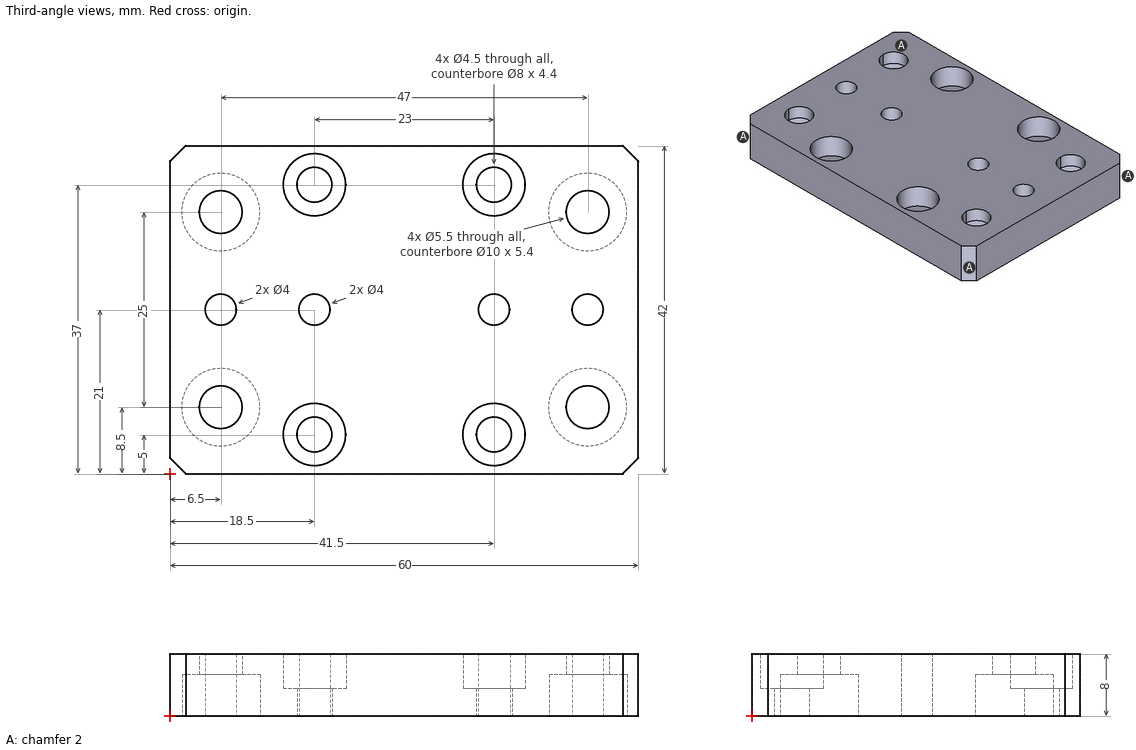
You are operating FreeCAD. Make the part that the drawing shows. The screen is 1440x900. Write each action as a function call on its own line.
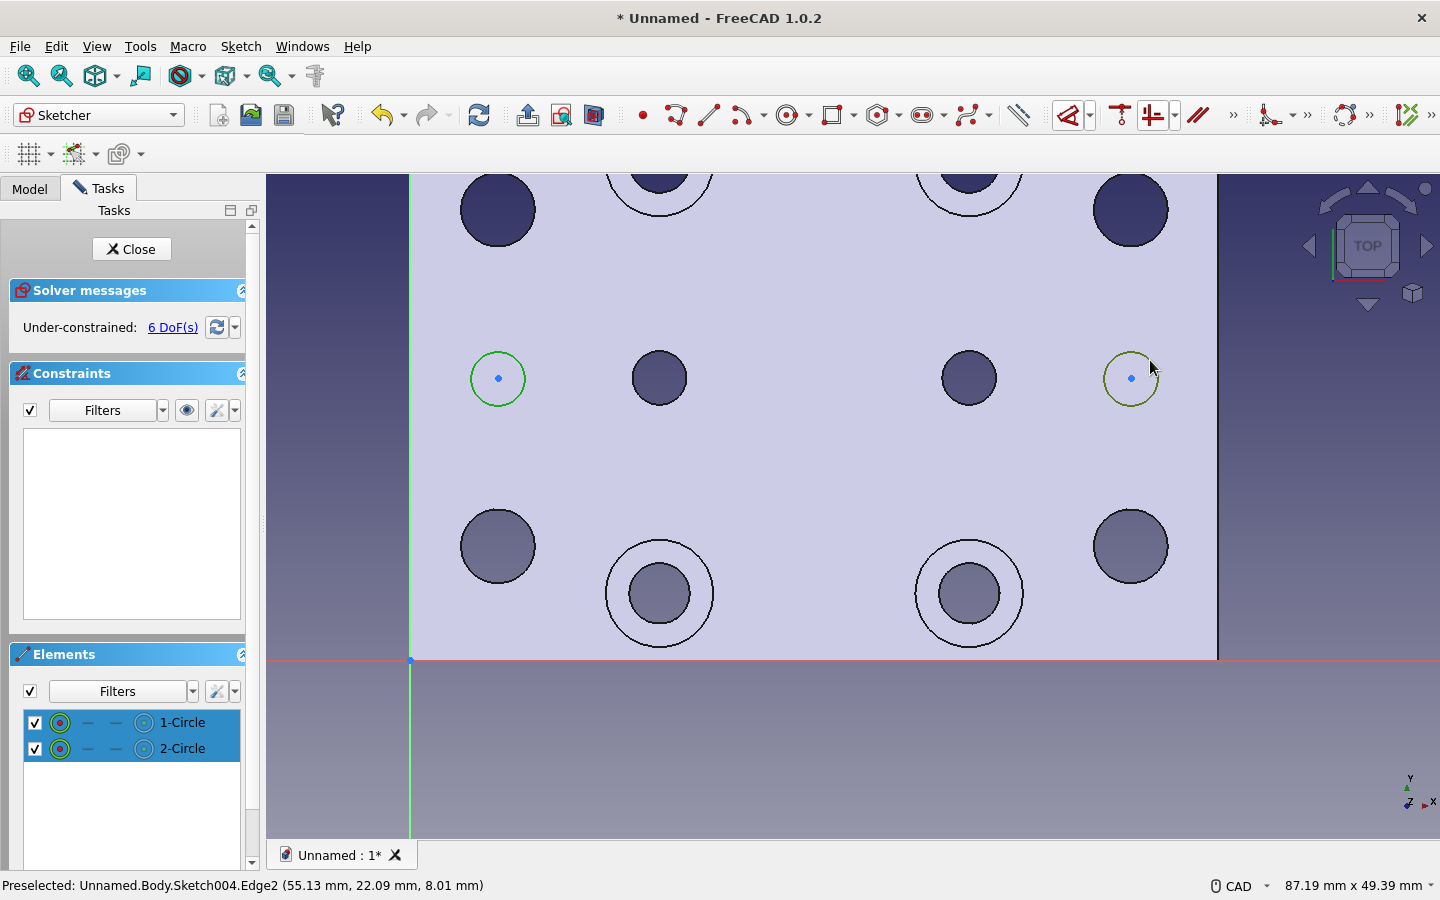
key(e)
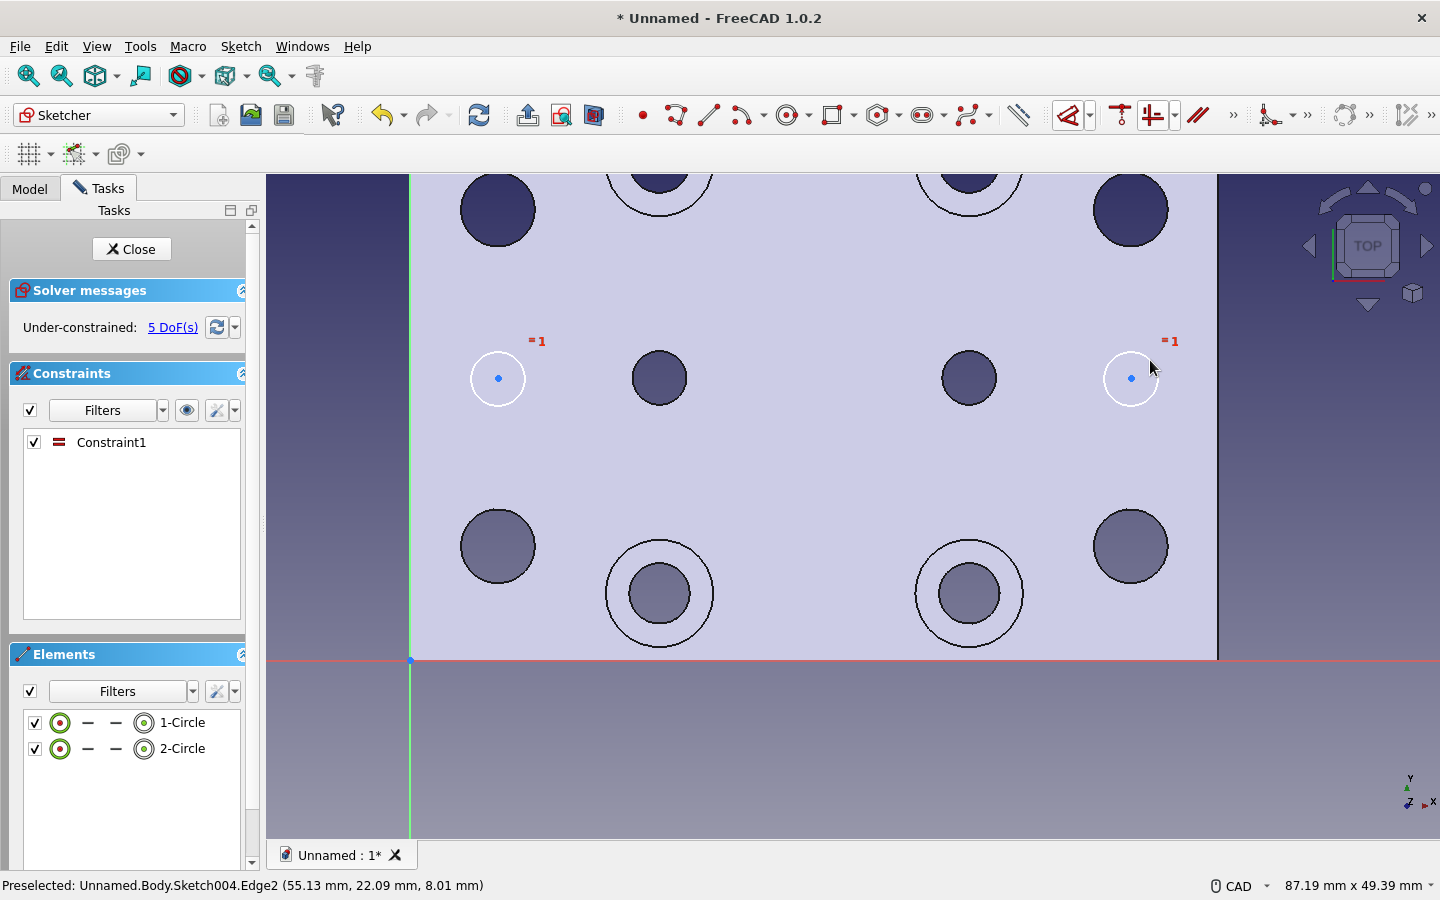
click(498, 379)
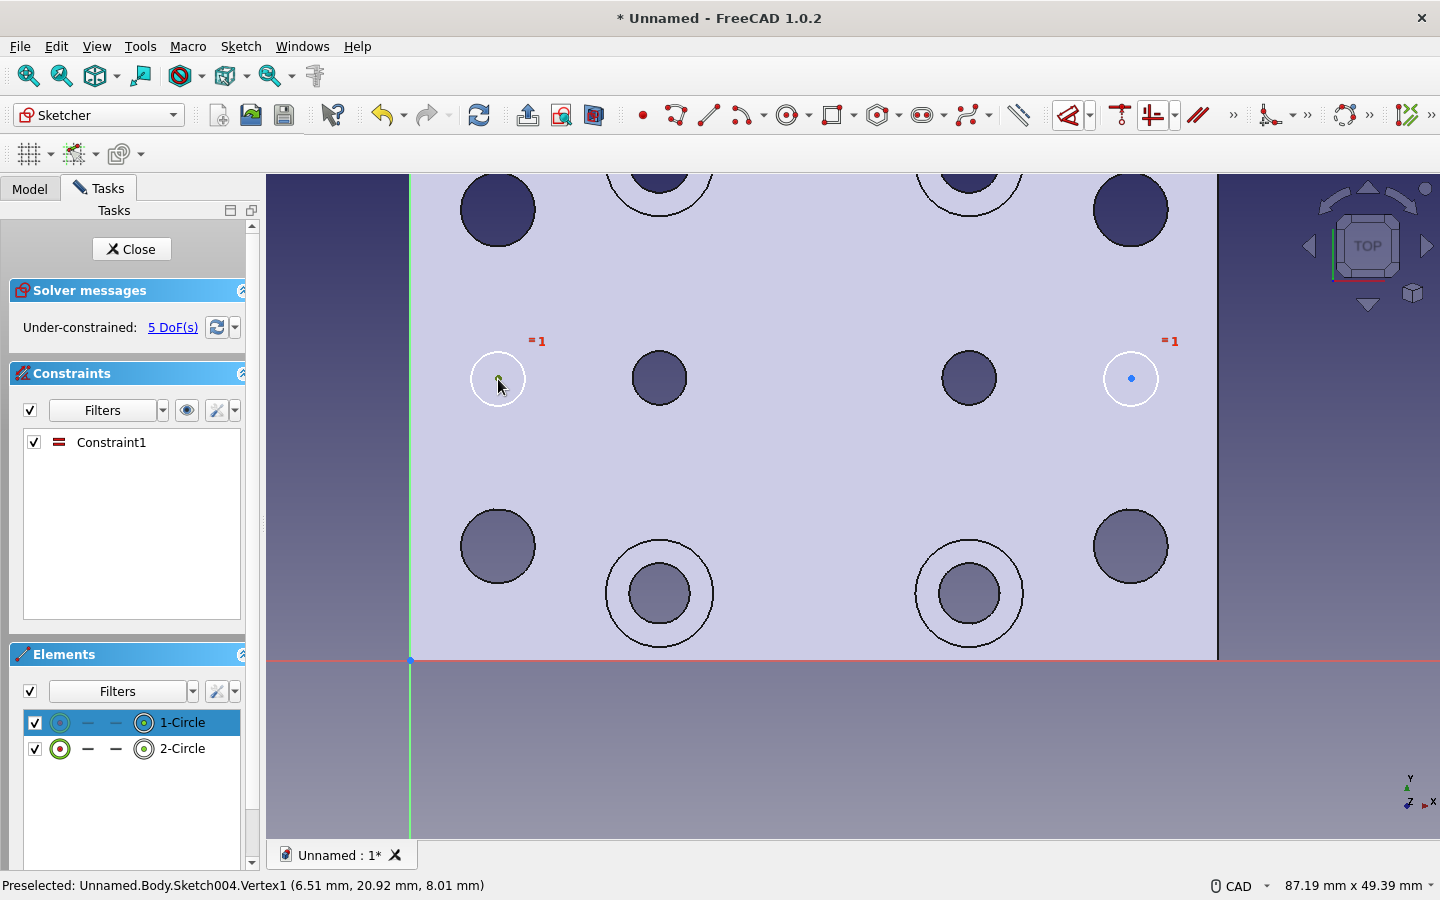
click(1131, 379)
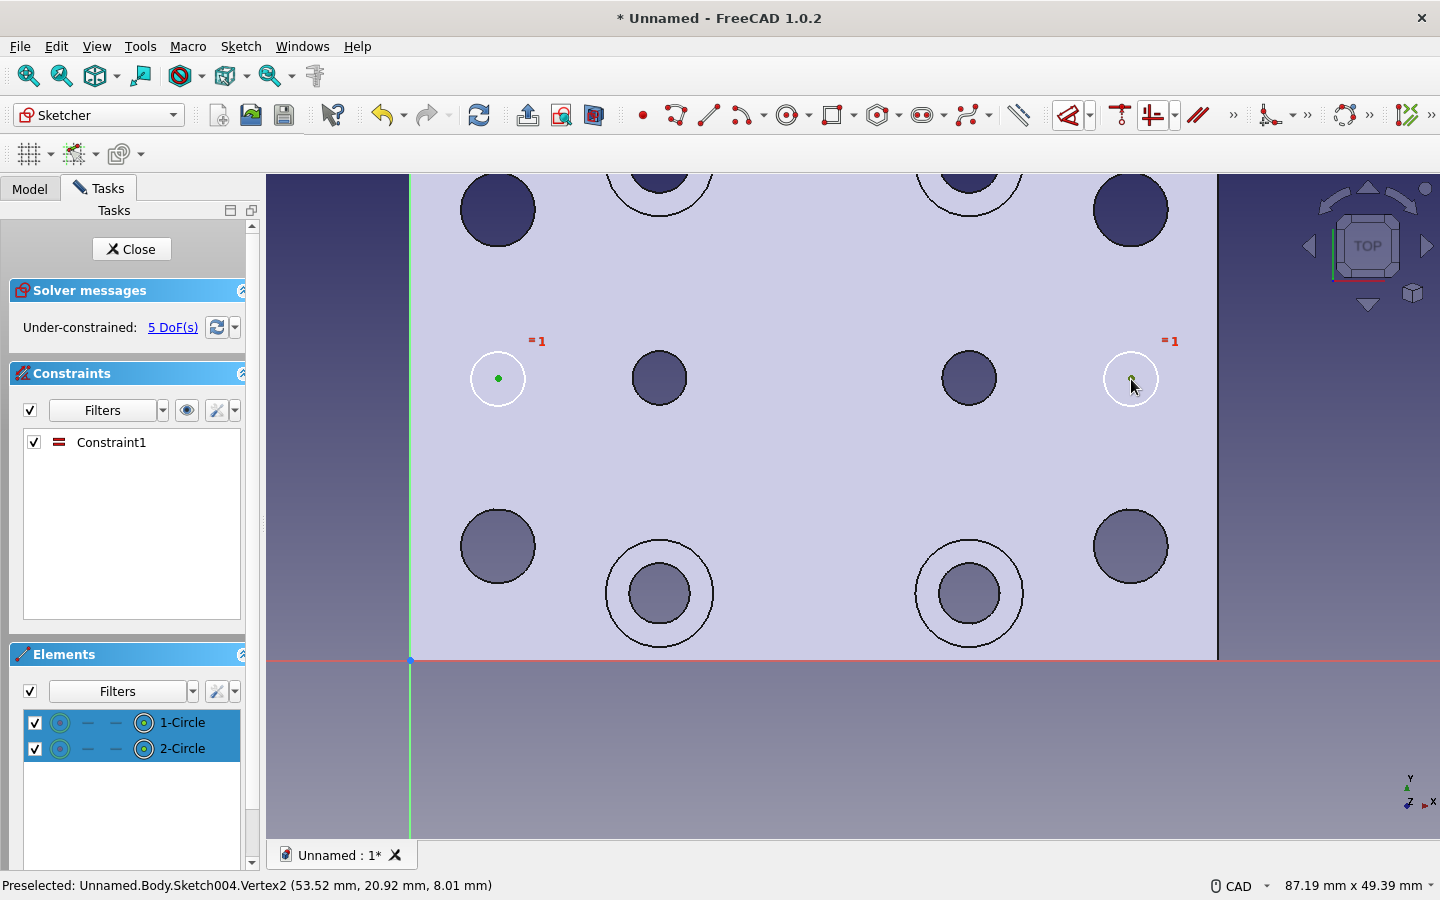
key(h)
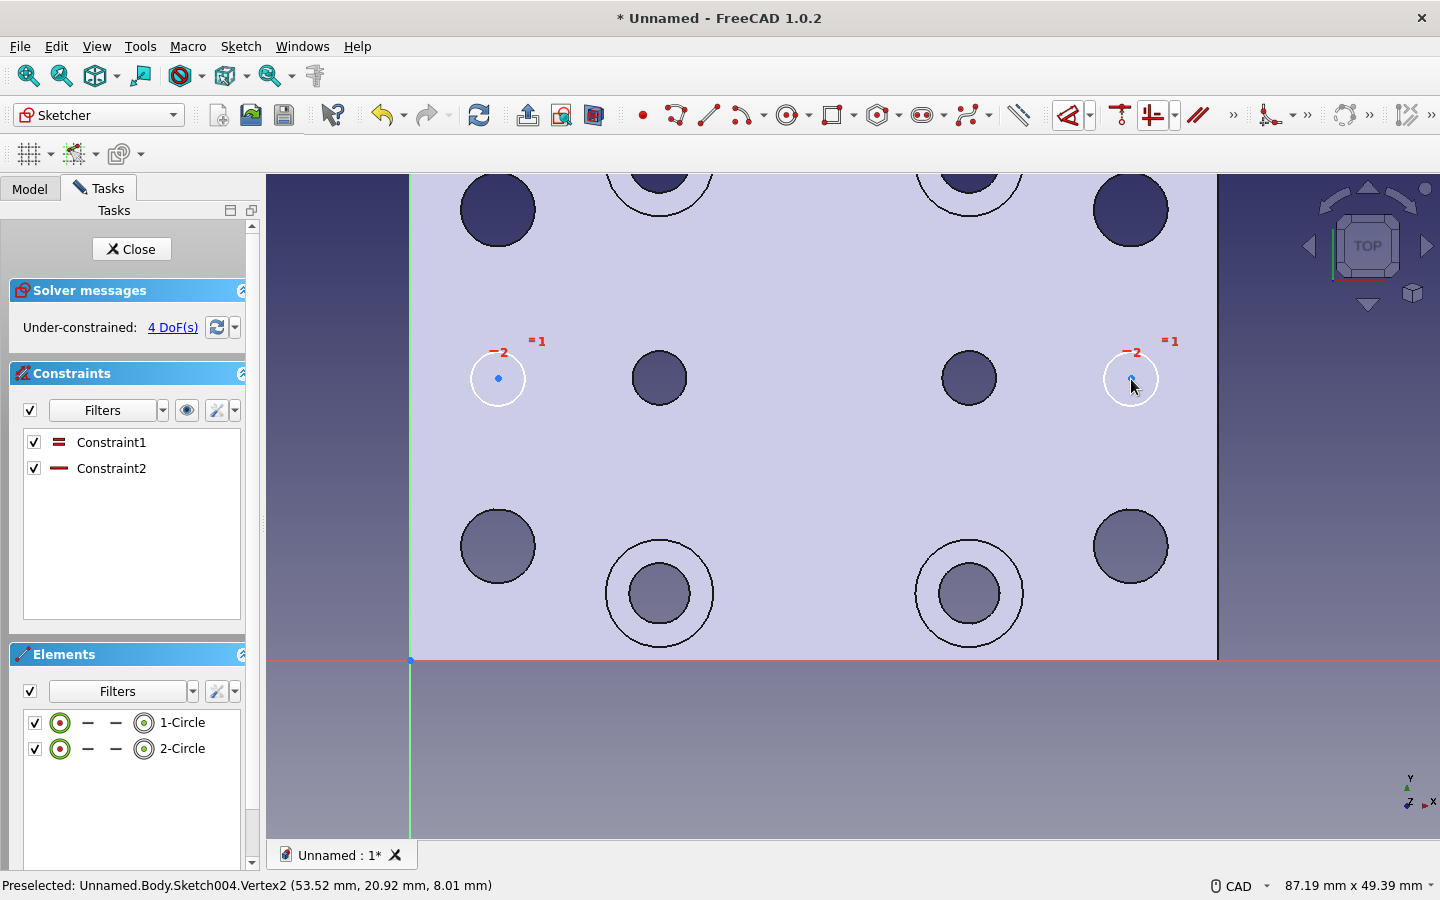
click(517, 360)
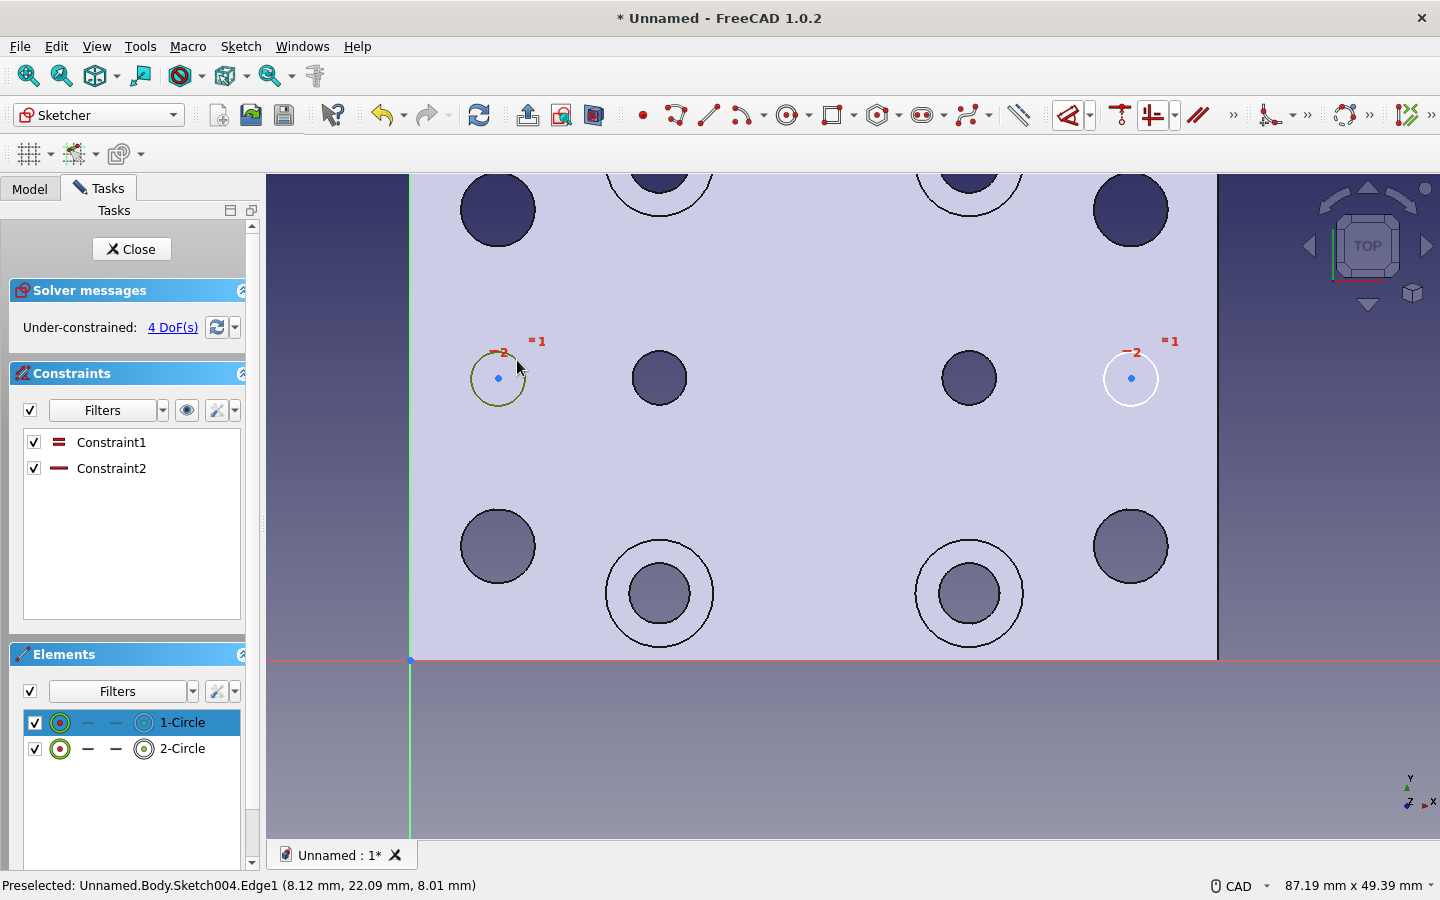
key(k)
key(o)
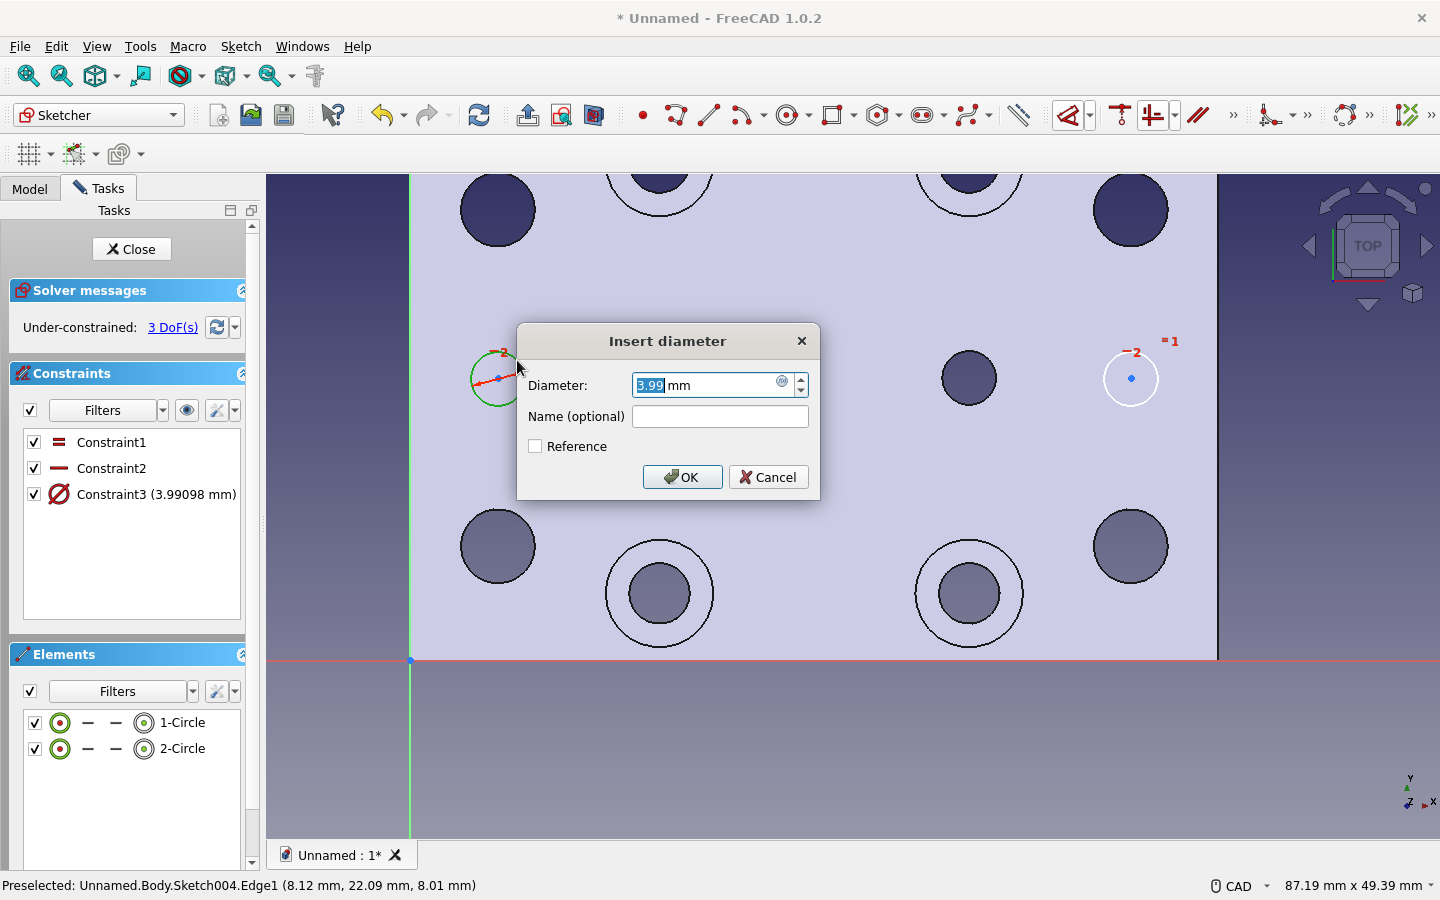
text(4)
key(Return)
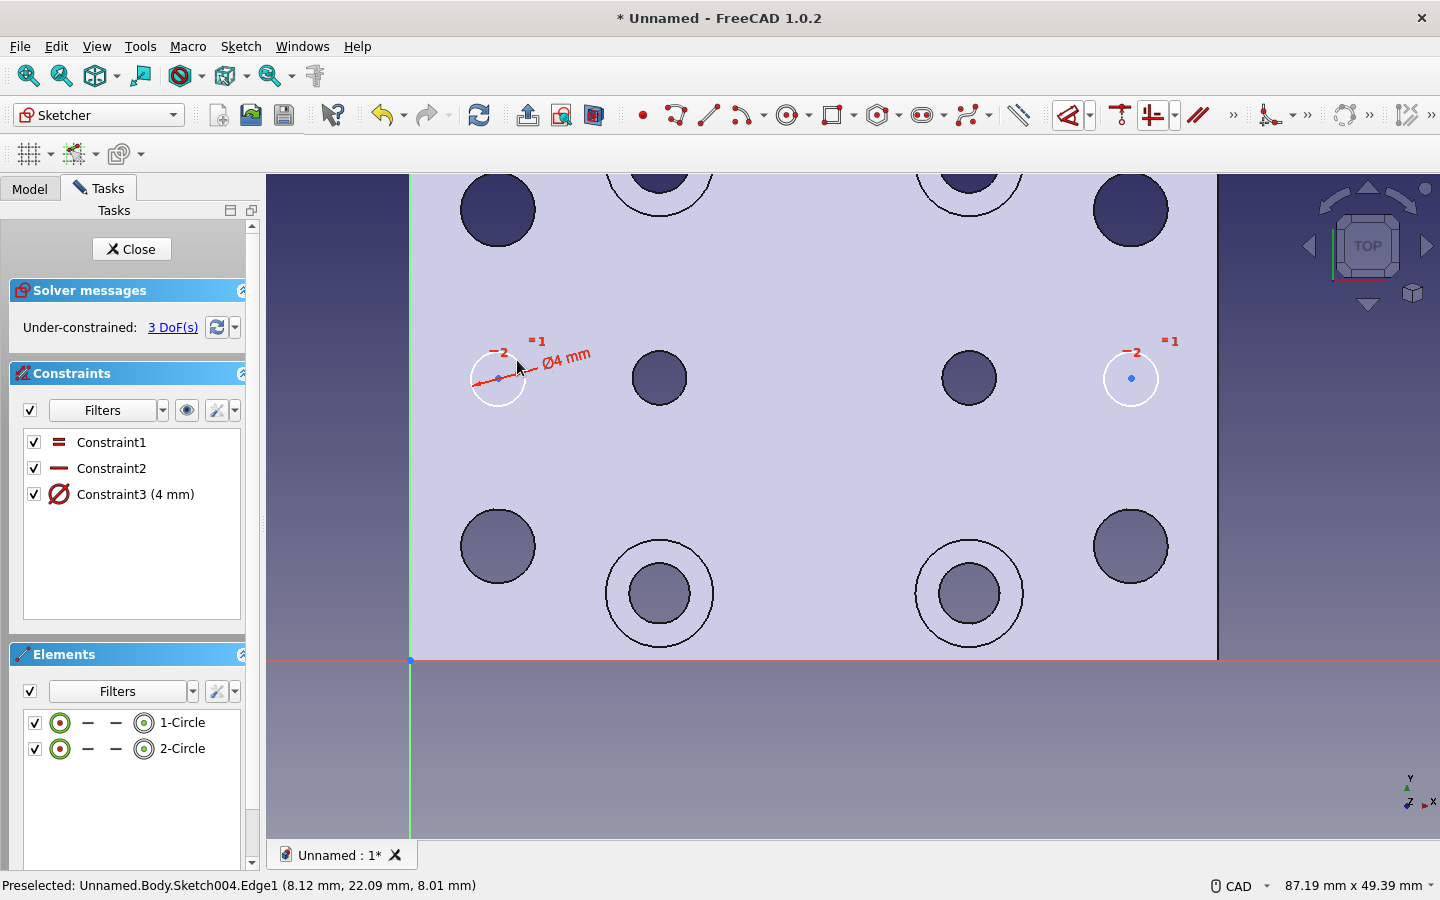
click(498, 379)